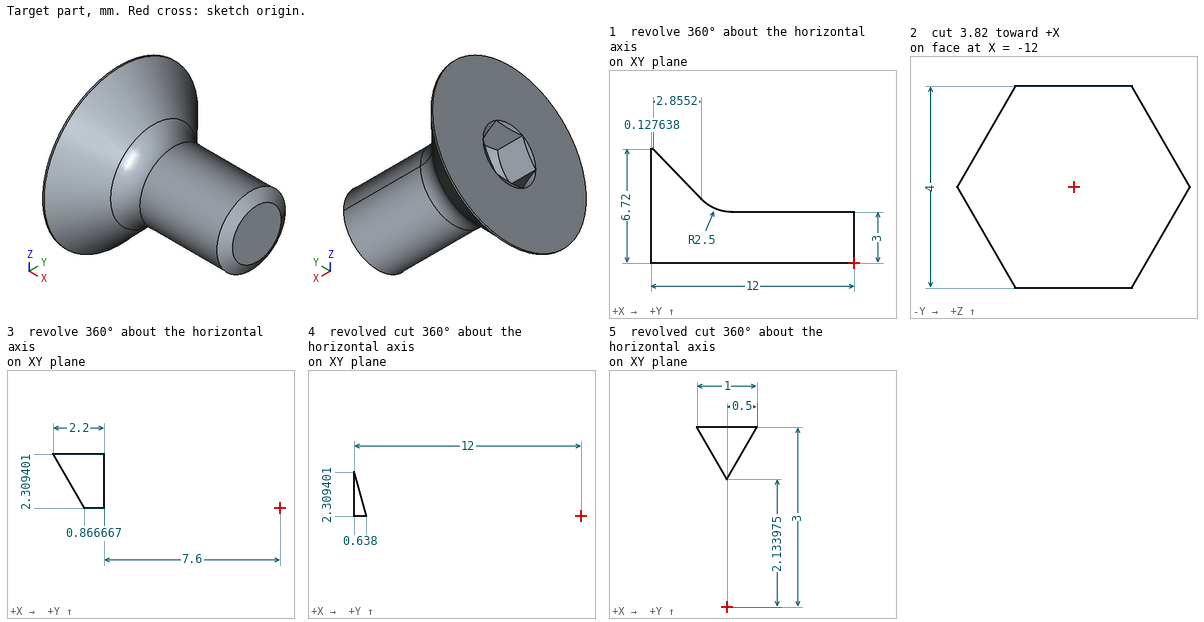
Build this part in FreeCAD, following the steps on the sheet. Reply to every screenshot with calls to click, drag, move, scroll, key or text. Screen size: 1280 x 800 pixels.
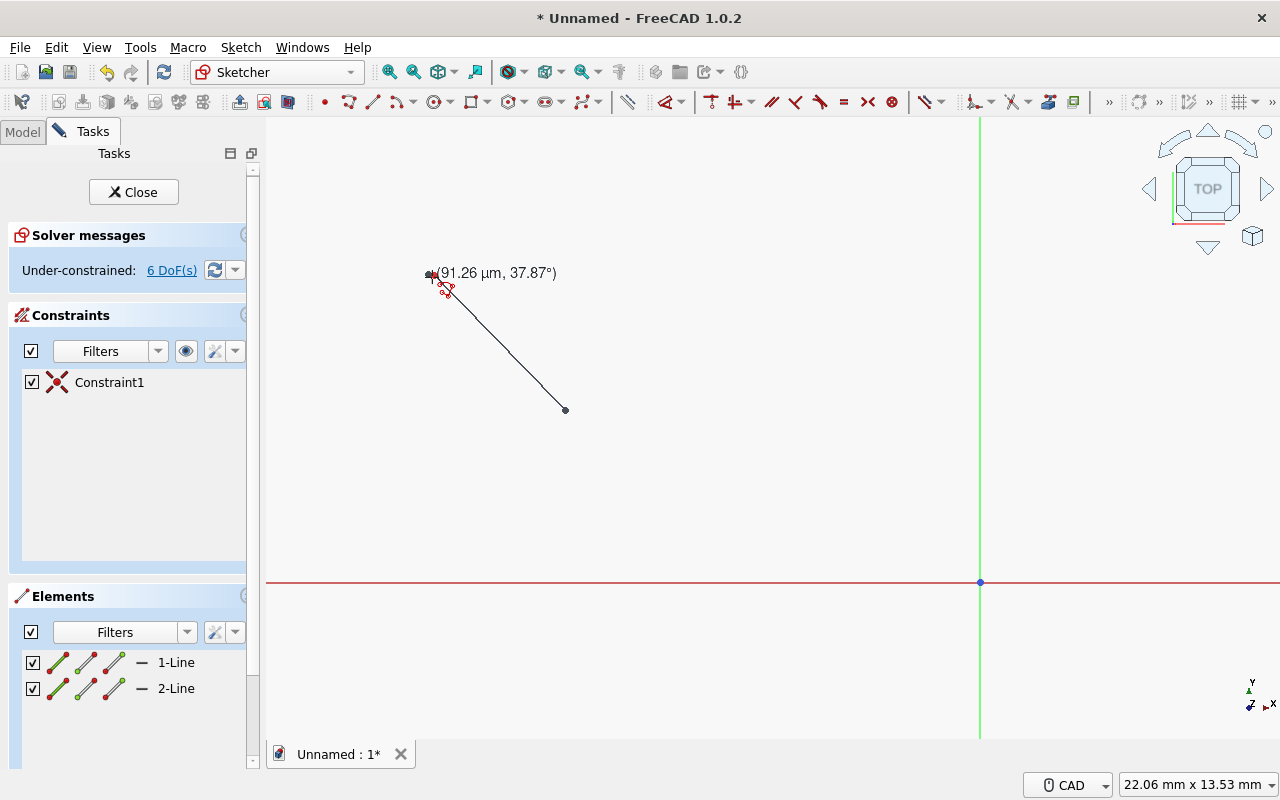
click(429, 583)
click(980, 583)
click(971, 445)
click(648, 445)
right_click(648, 445)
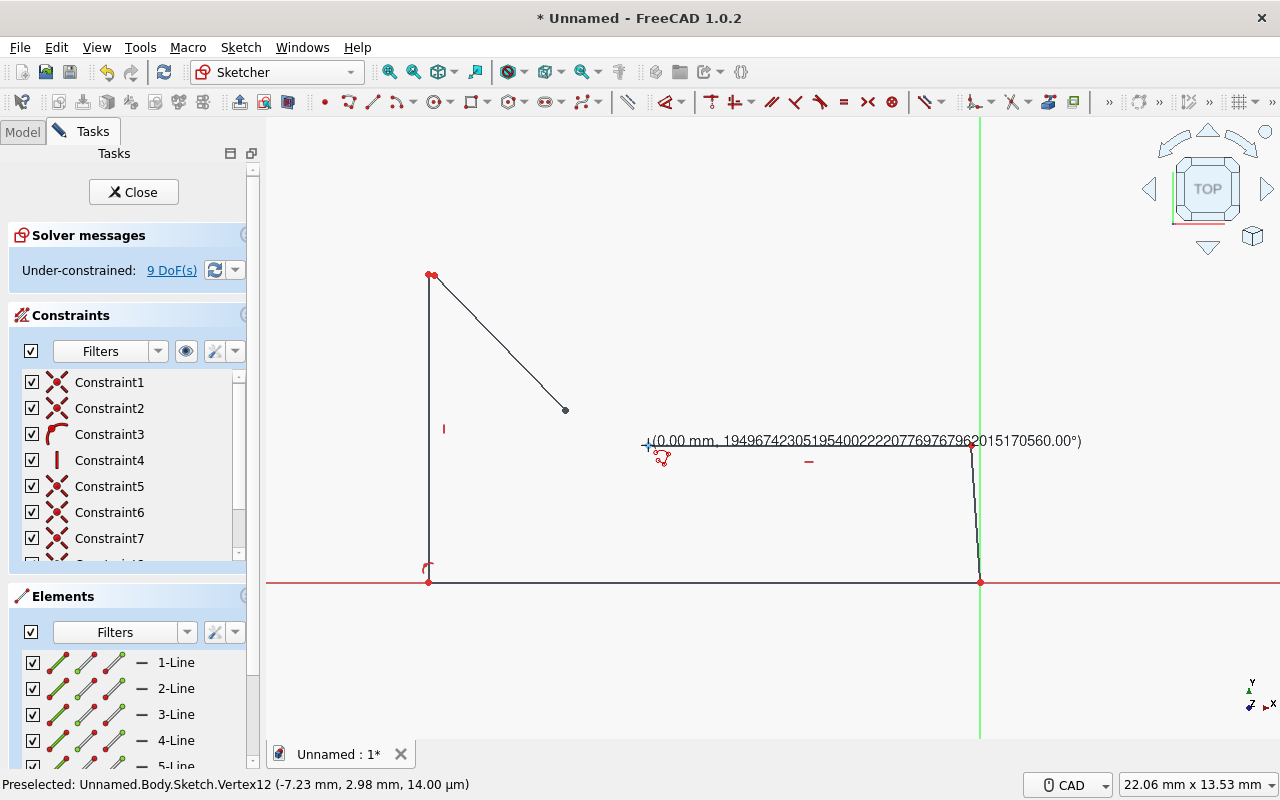
key(g)
key(3)
key(a)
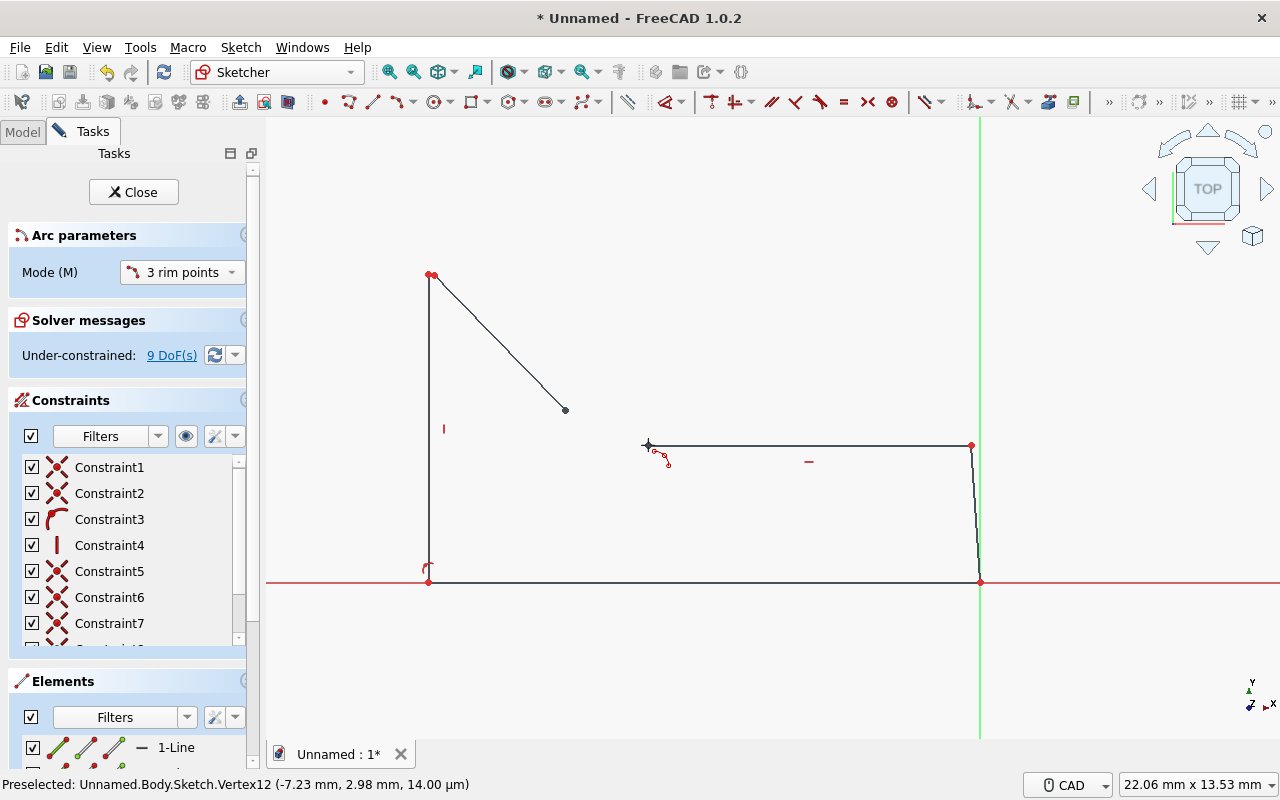
click(648, 446)
click(566, 410)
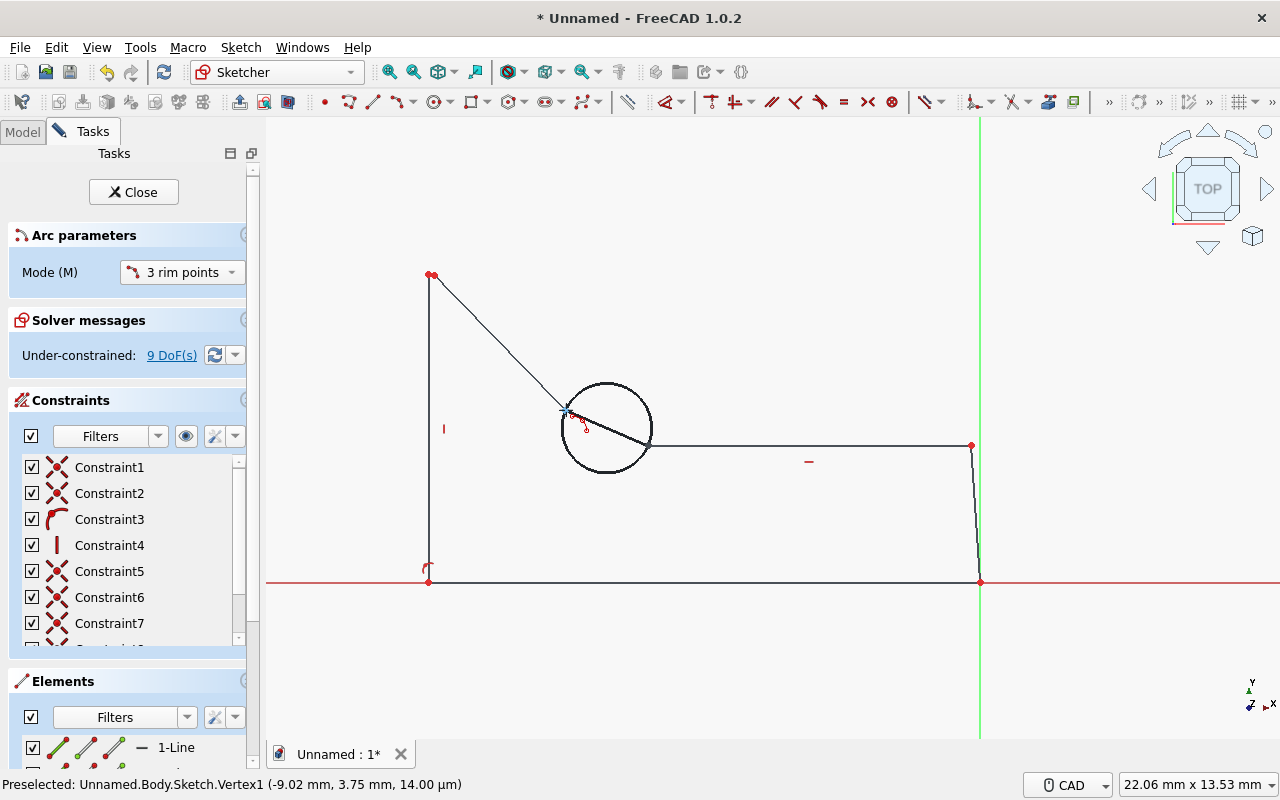
scroll(603, 436, up, 3)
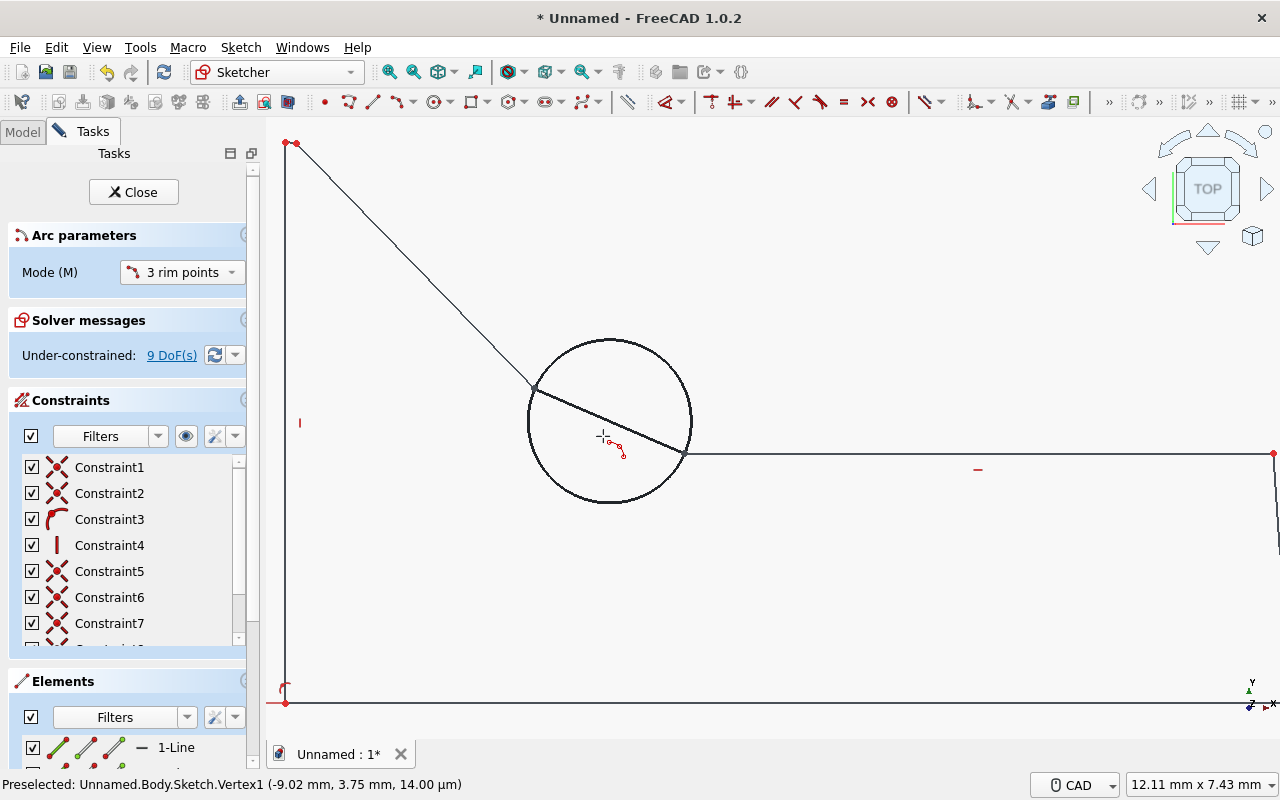
click(604, 435)
key(Escape)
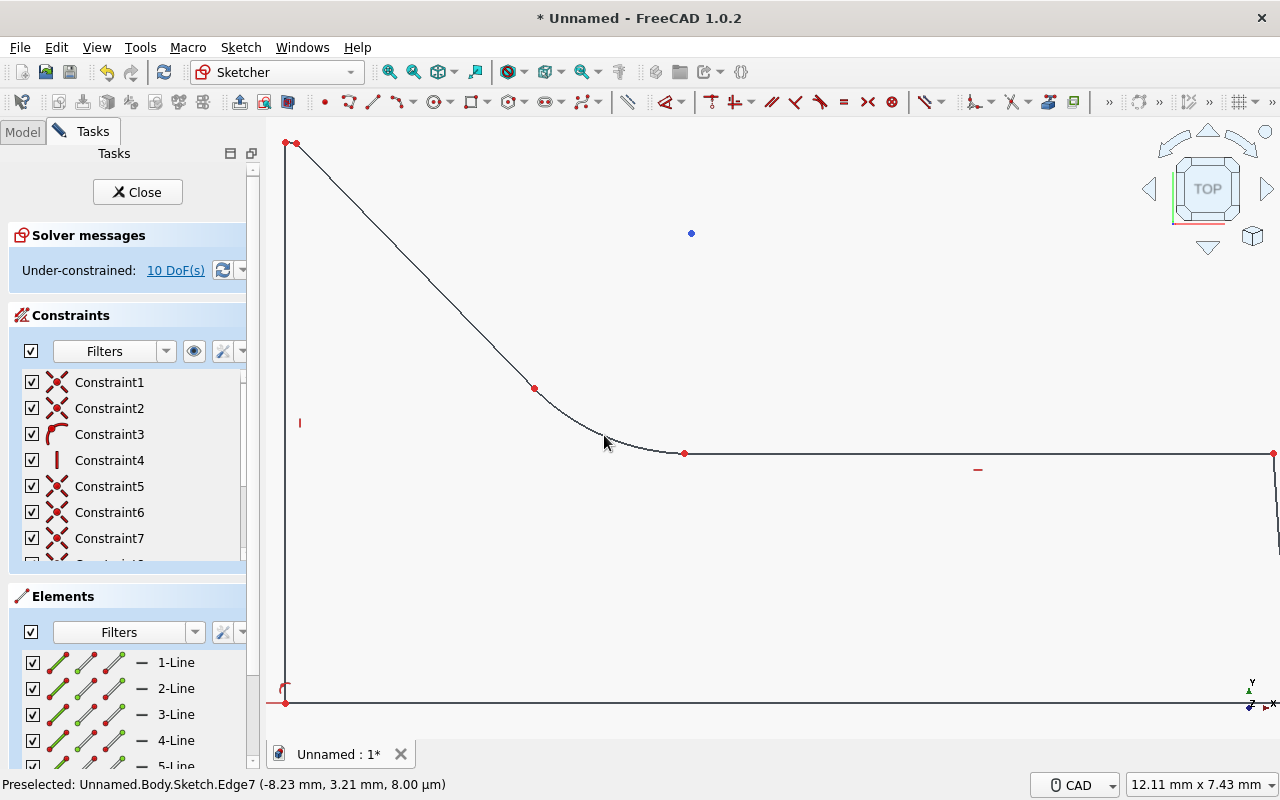
click(463, 315)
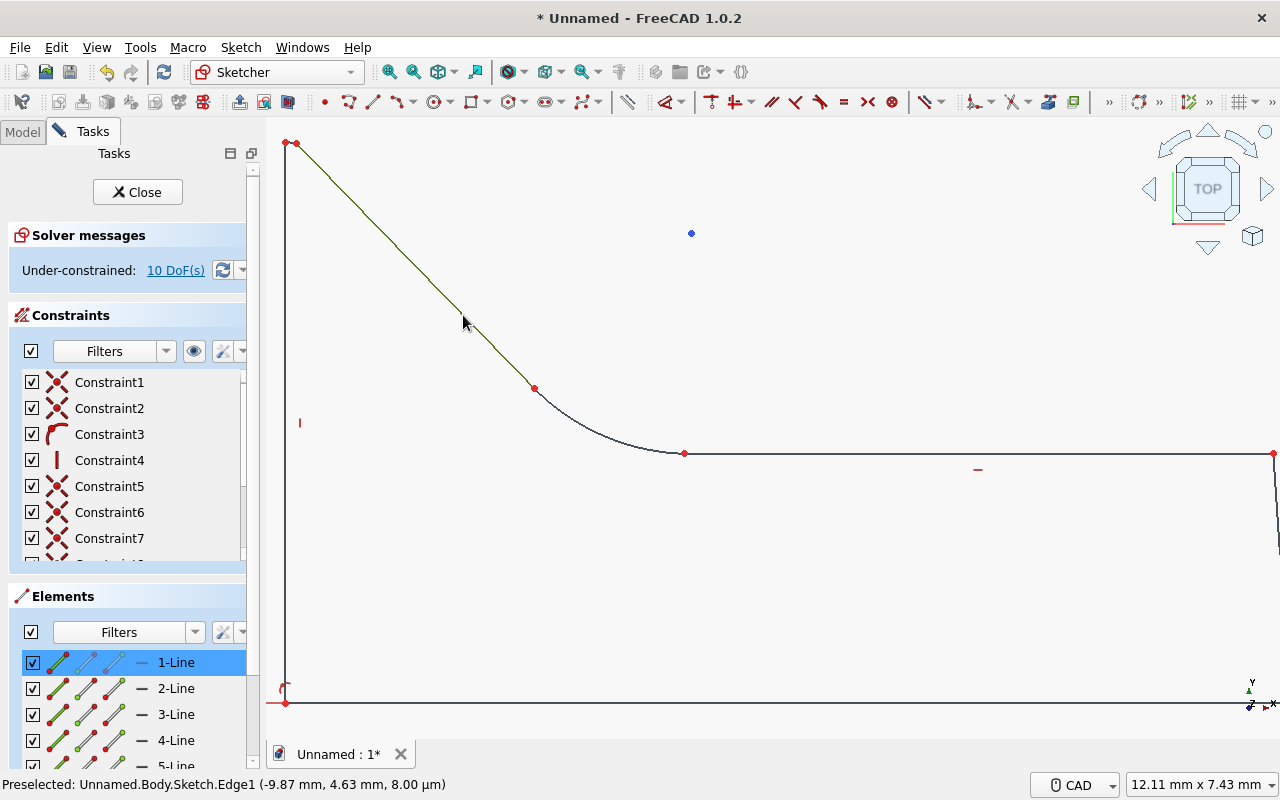
click(574, 420)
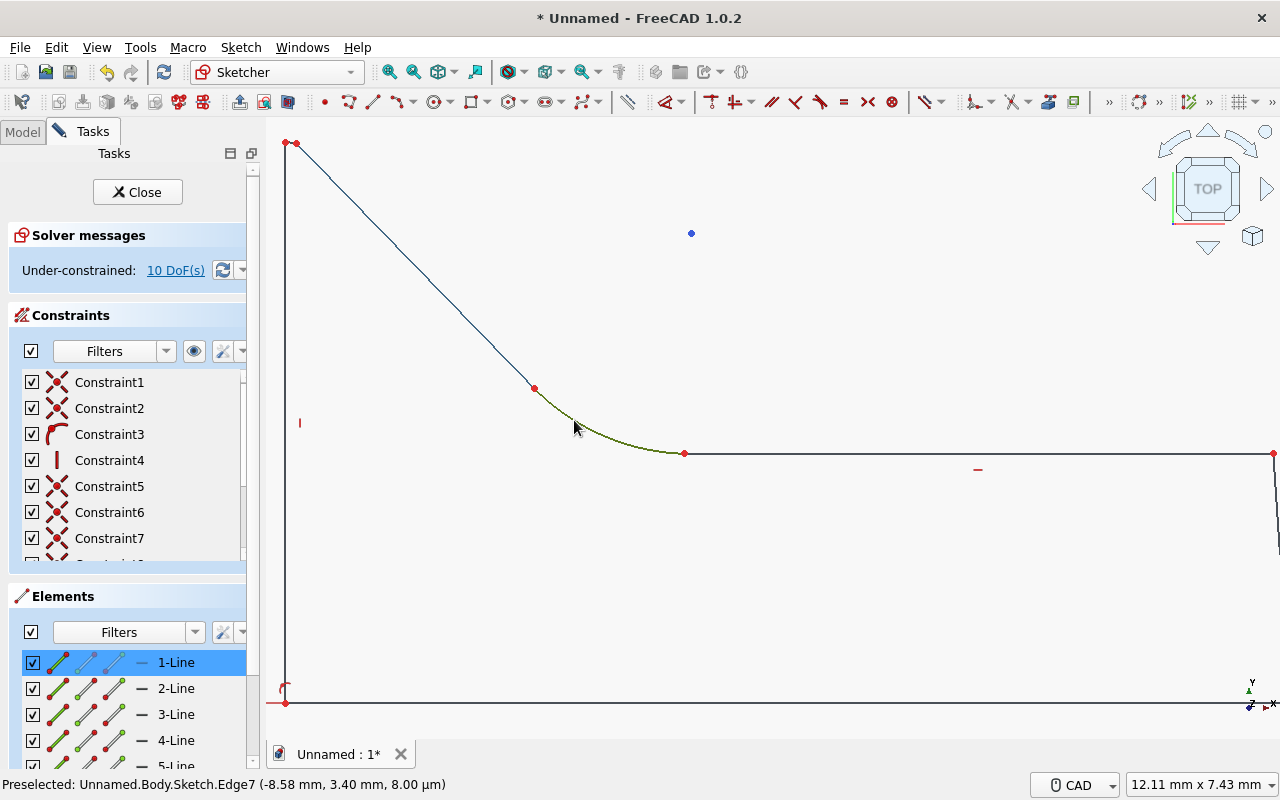
key(t)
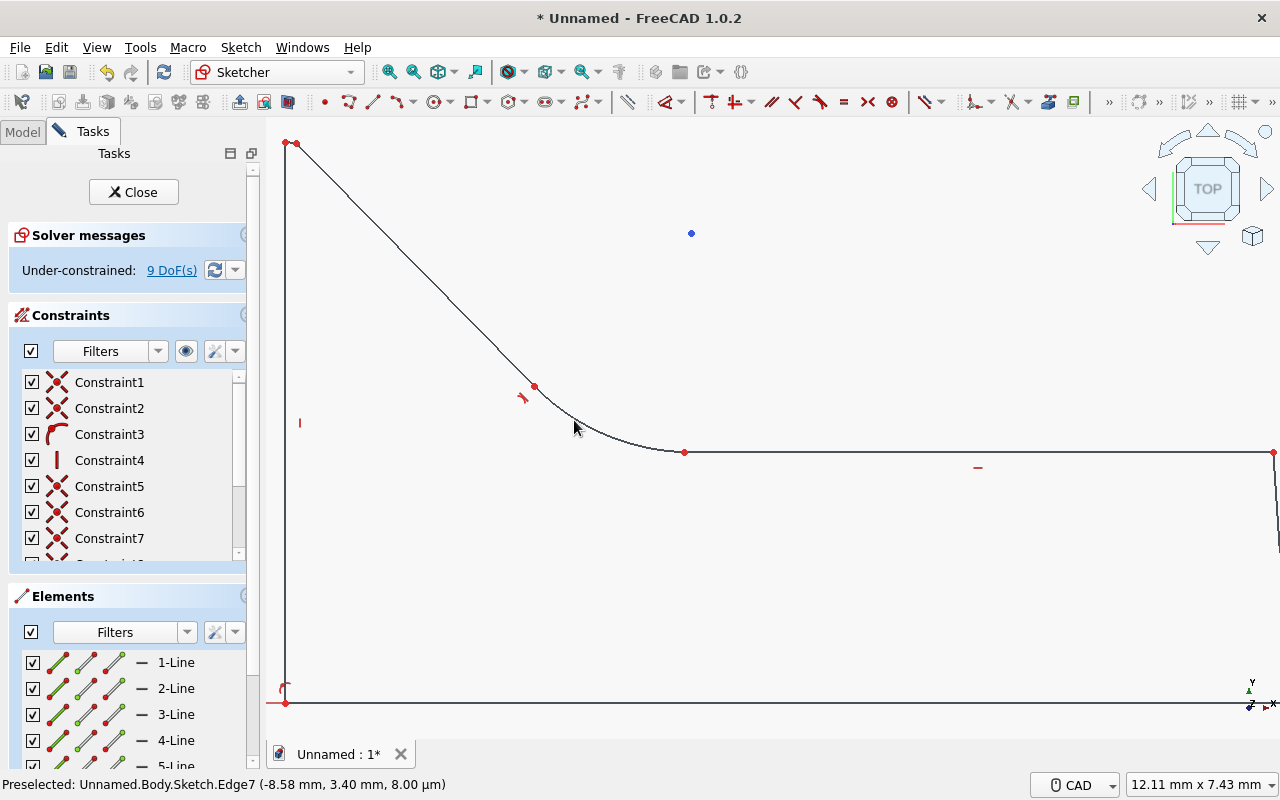
click(1097, 452)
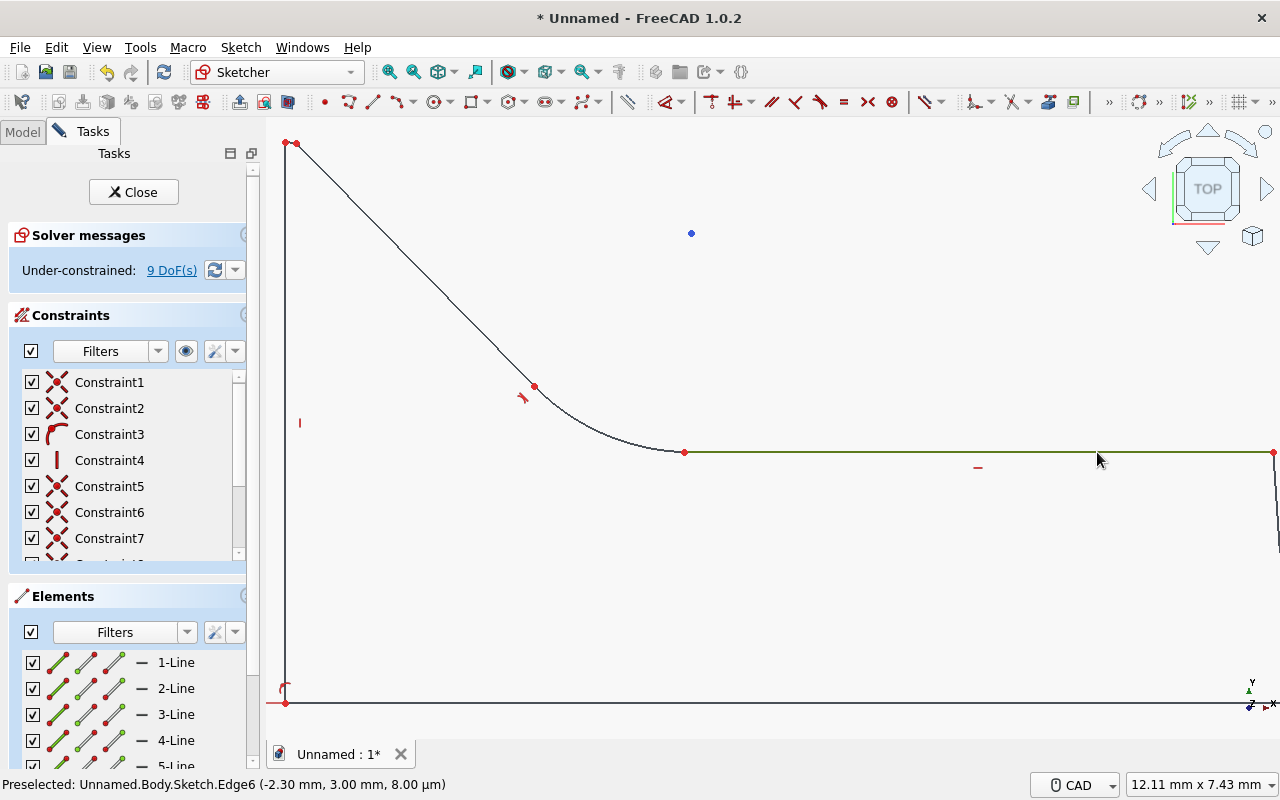
click(574, 418)